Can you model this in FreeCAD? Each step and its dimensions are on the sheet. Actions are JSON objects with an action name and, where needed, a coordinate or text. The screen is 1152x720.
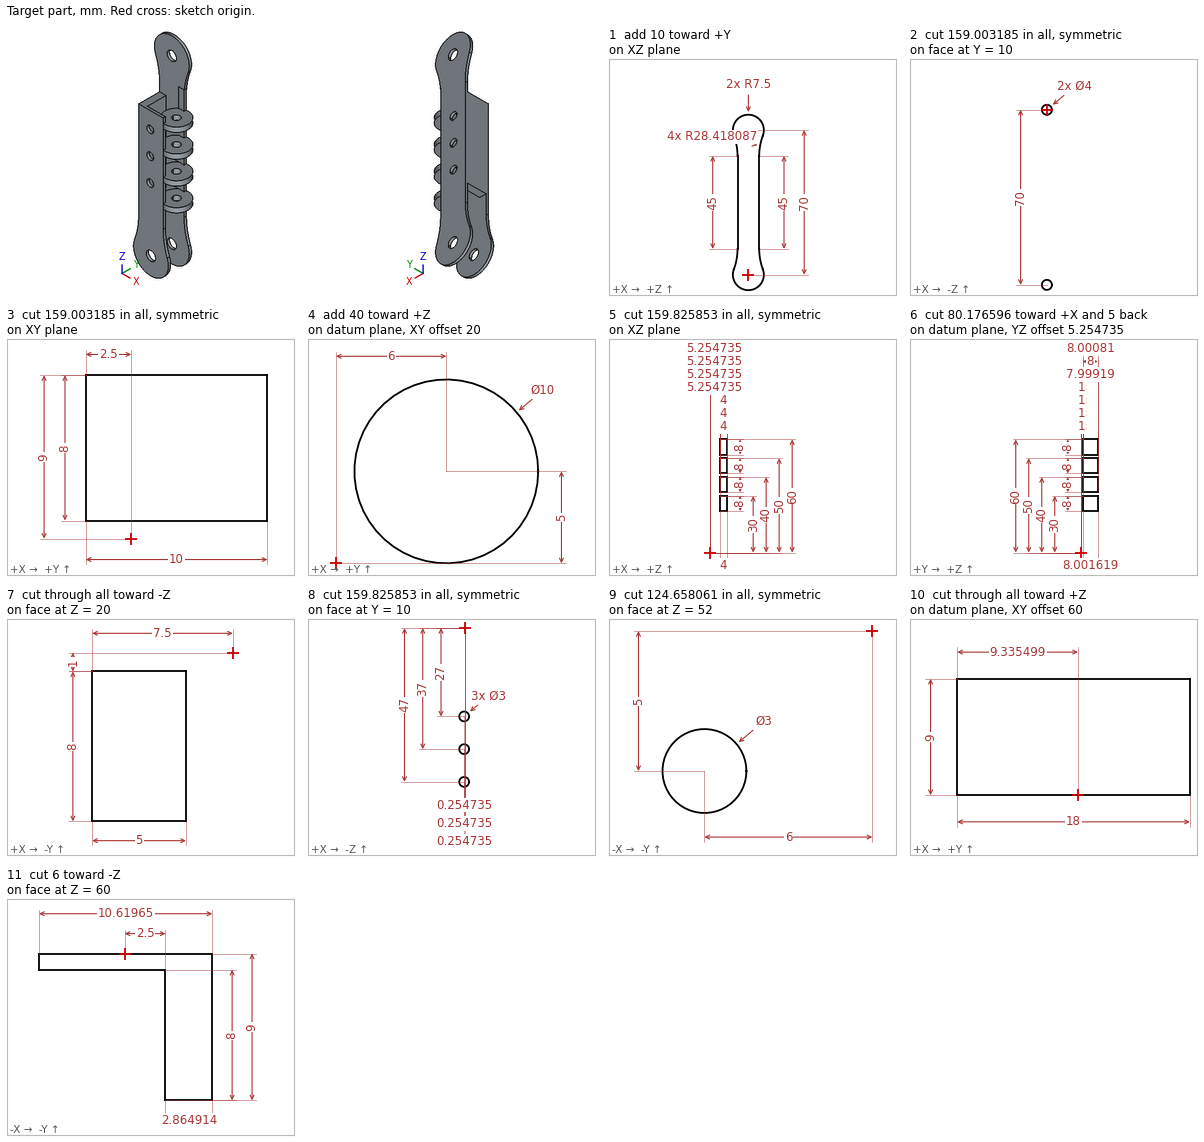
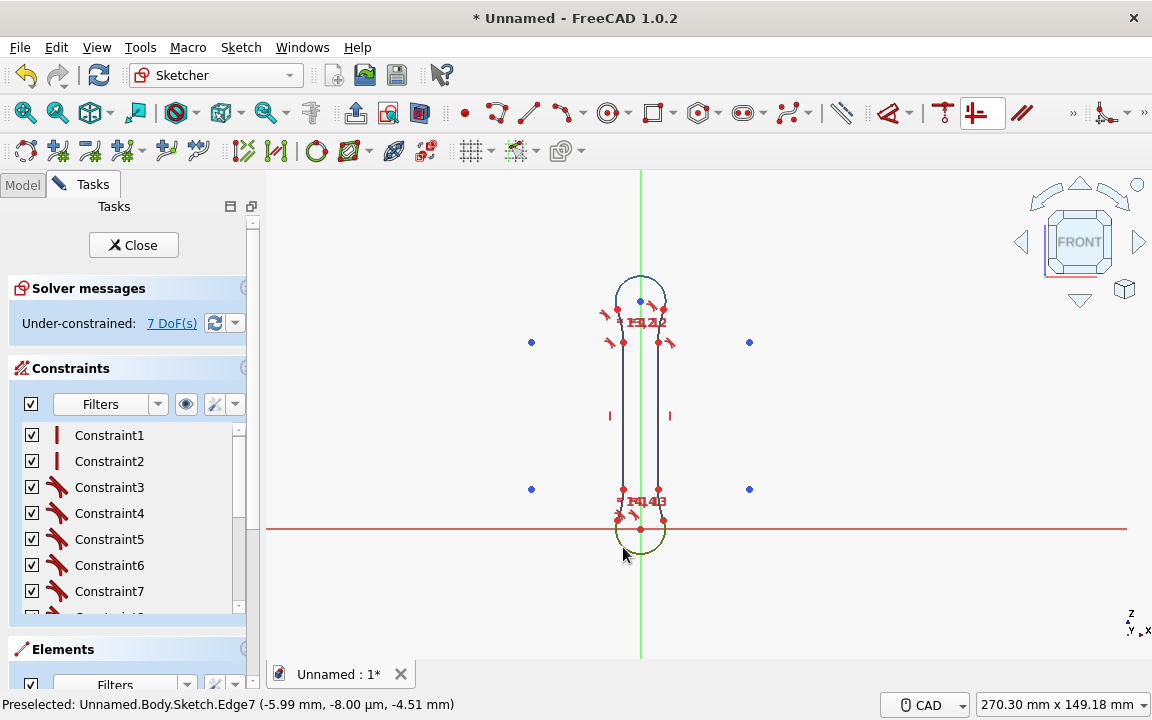
{"action": "key", "text": "e"}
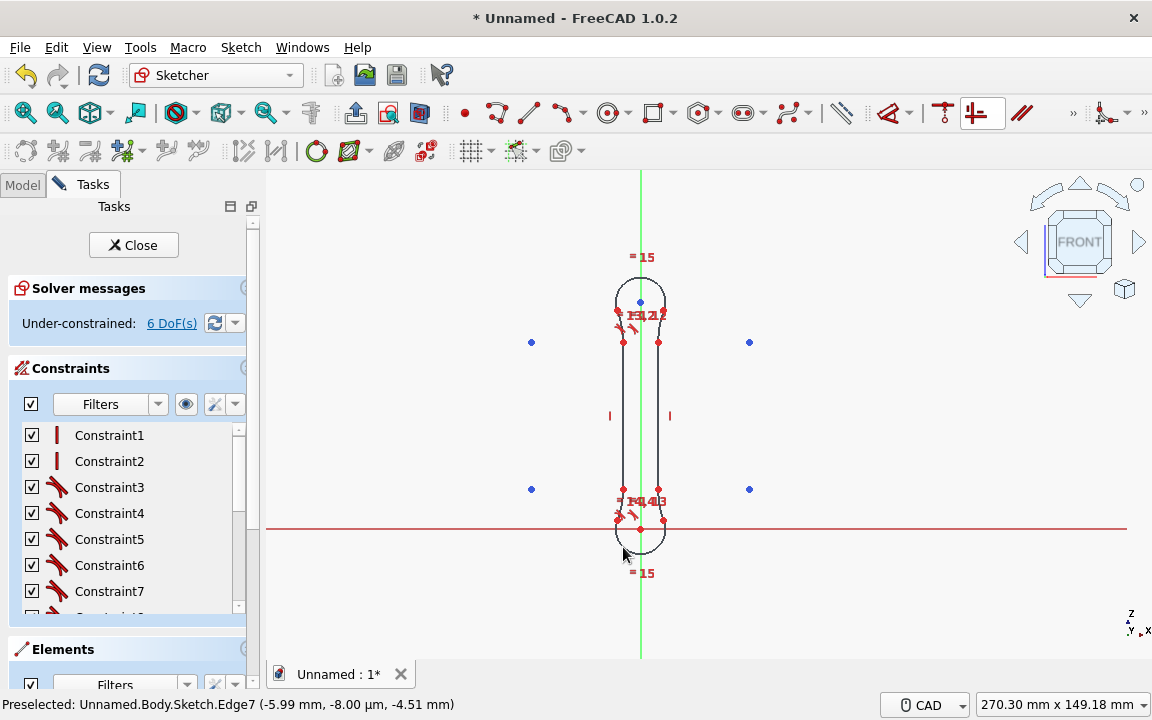
{"action": "left_click", "coordinate": [641, 302]}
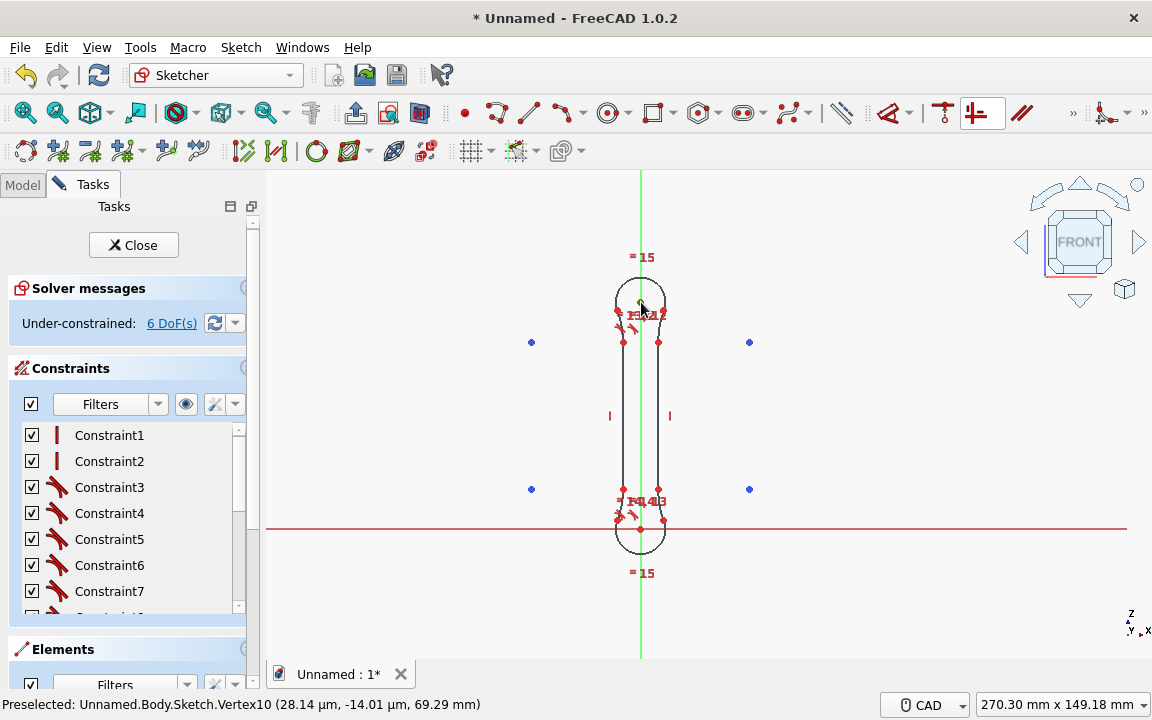
{"action": "left_click", "coordinate": [641, 600]}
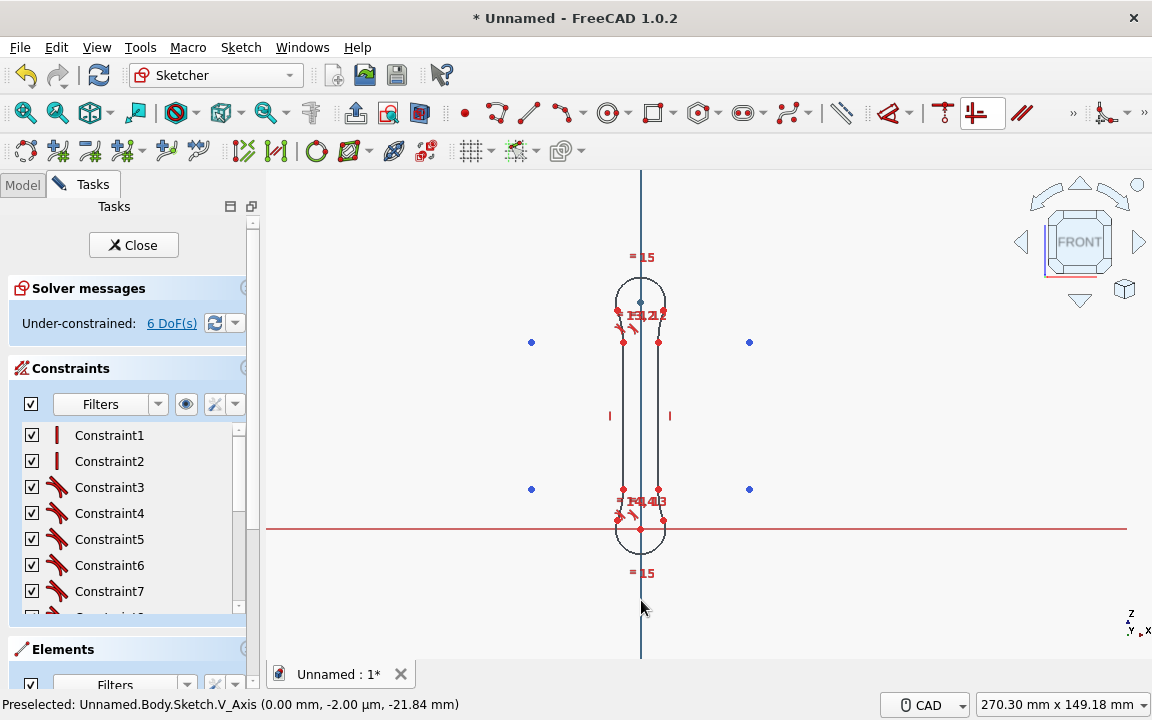
{"action": "left_click", "coordinate": [944, 114]}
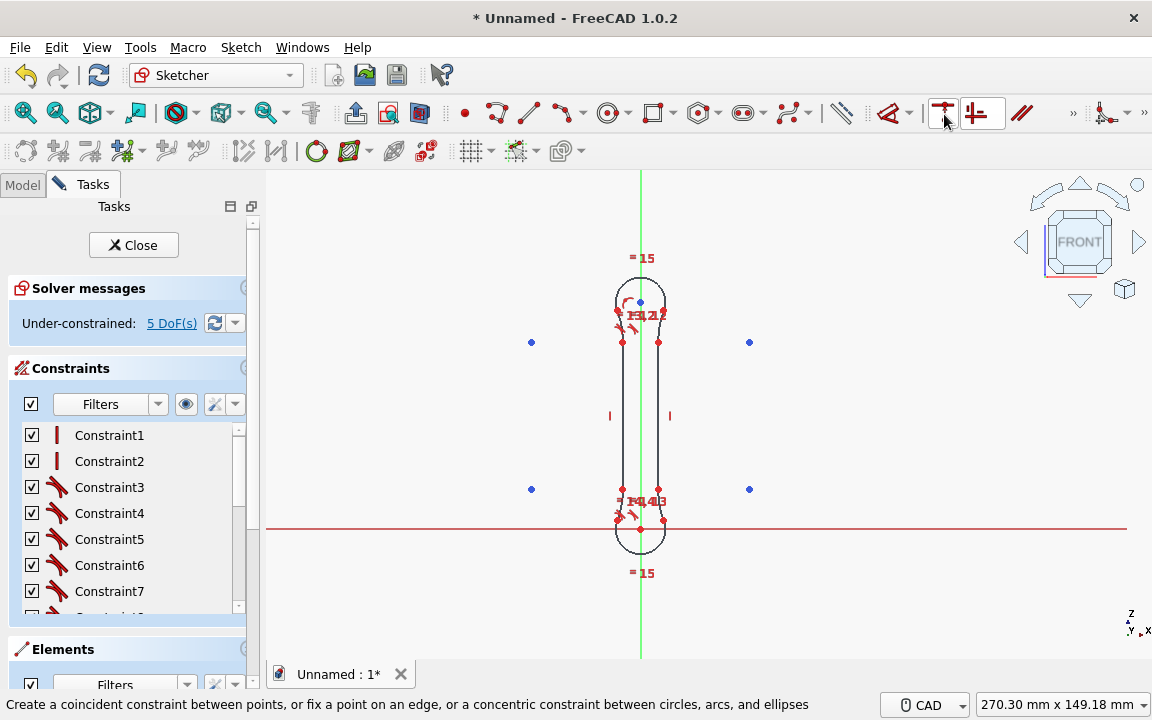
{"action": "left_click", "coordinate": [888, 114]}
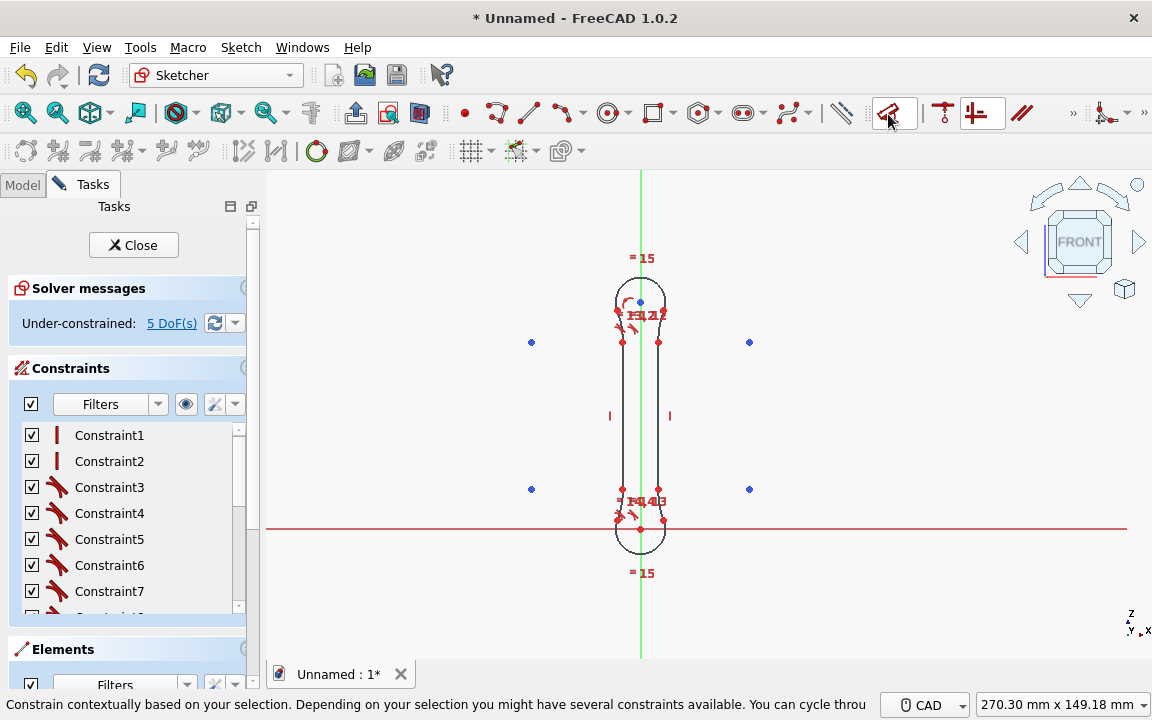
{"action": "scroll", "coordinate": [622, 333], "scroll_direction": "up", "scroll_amount": 2}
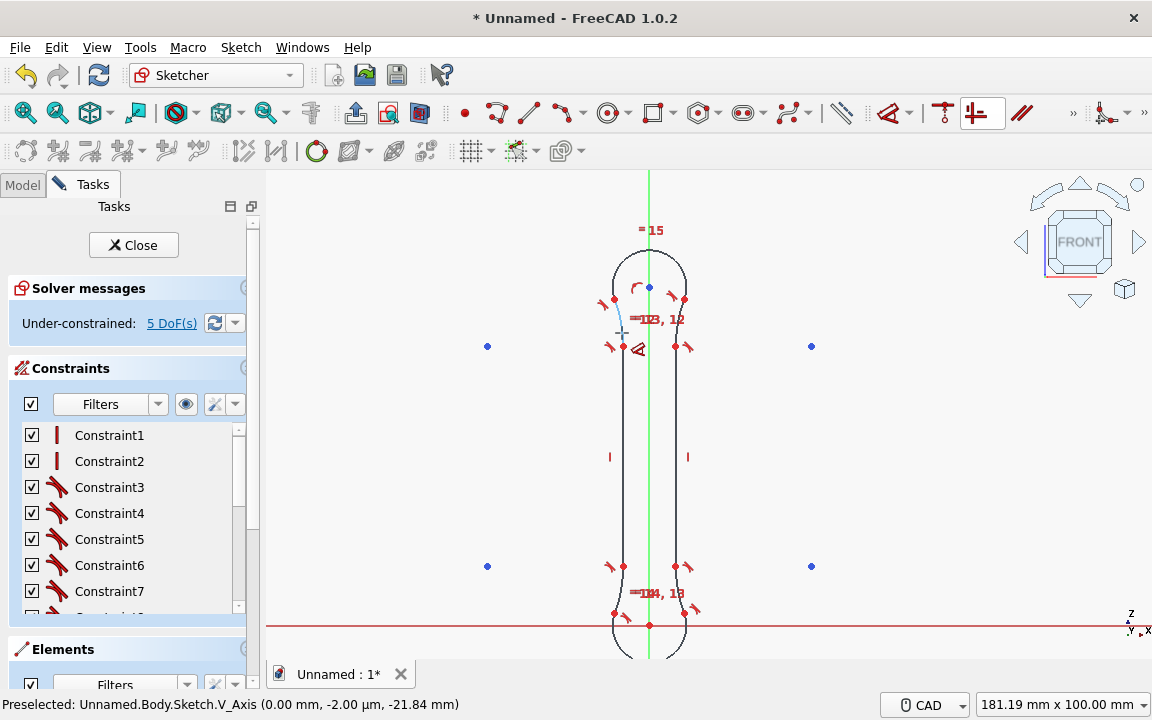
{"action": "left_click", "coordinate": [622, 332]}
{"action": "left_click", "coordinate": [592, 477]}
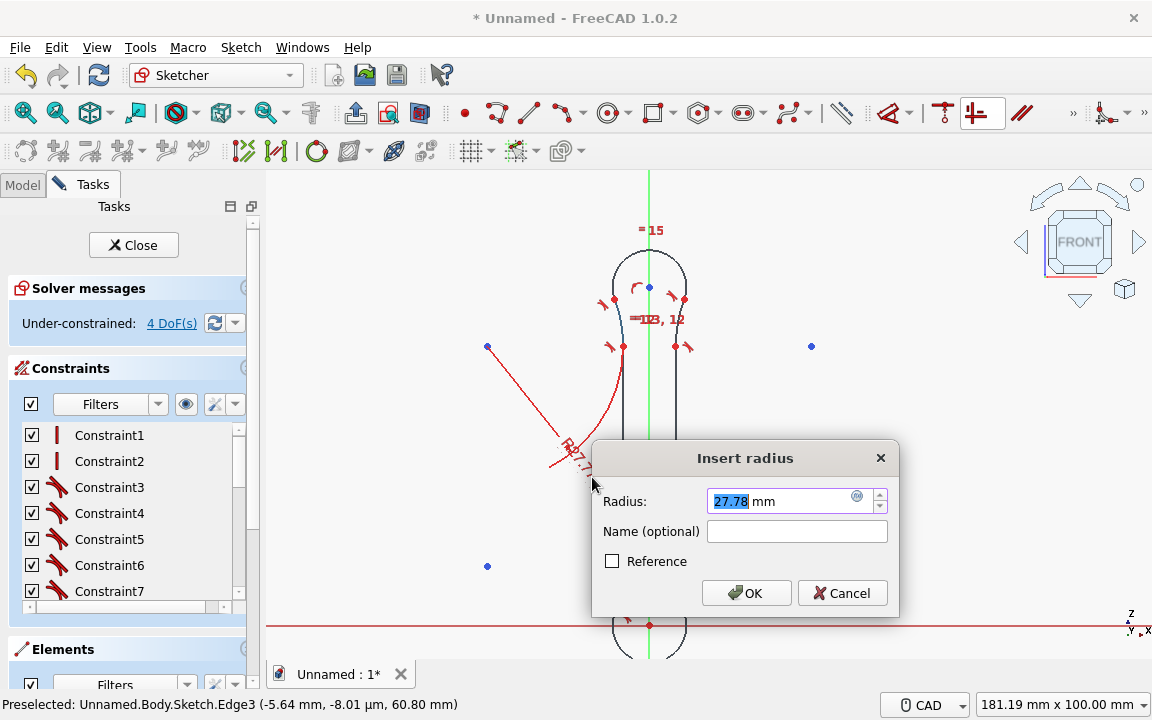
{"action": "type", "text": "28.418087"}
{"action": "key", "text": "Return"}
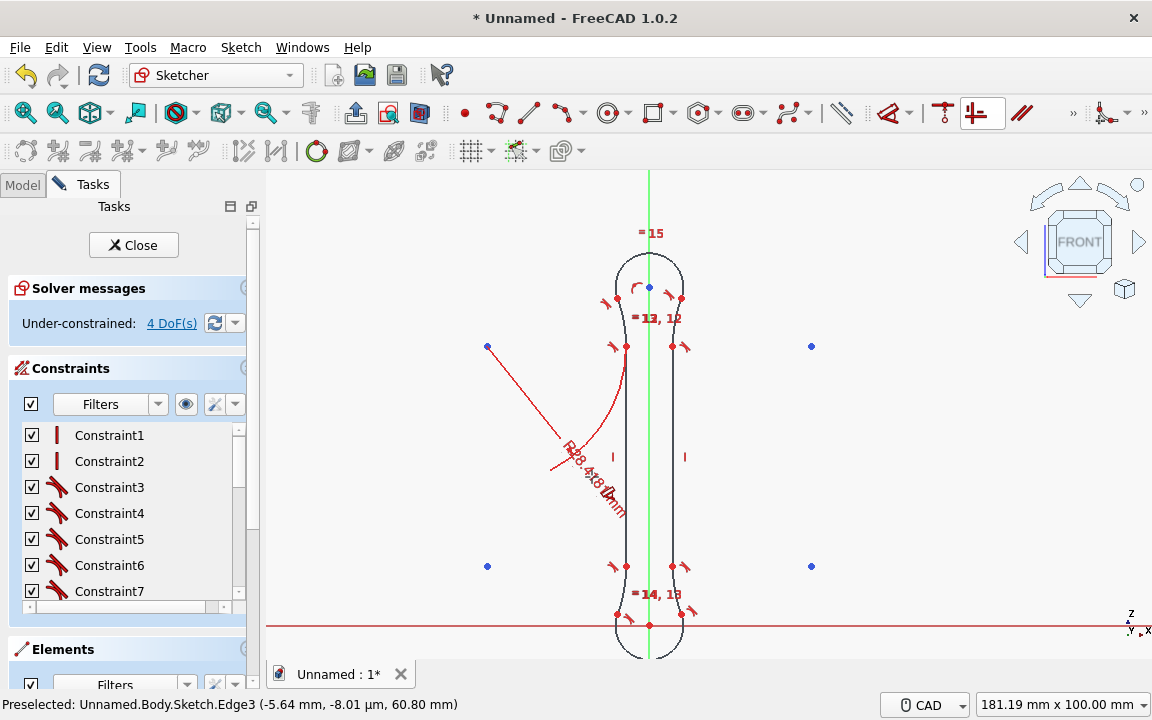
{"action": "left_click", "coordinate": [673, 263]}
{"action": "left_click", "coordinate": [695, 240]}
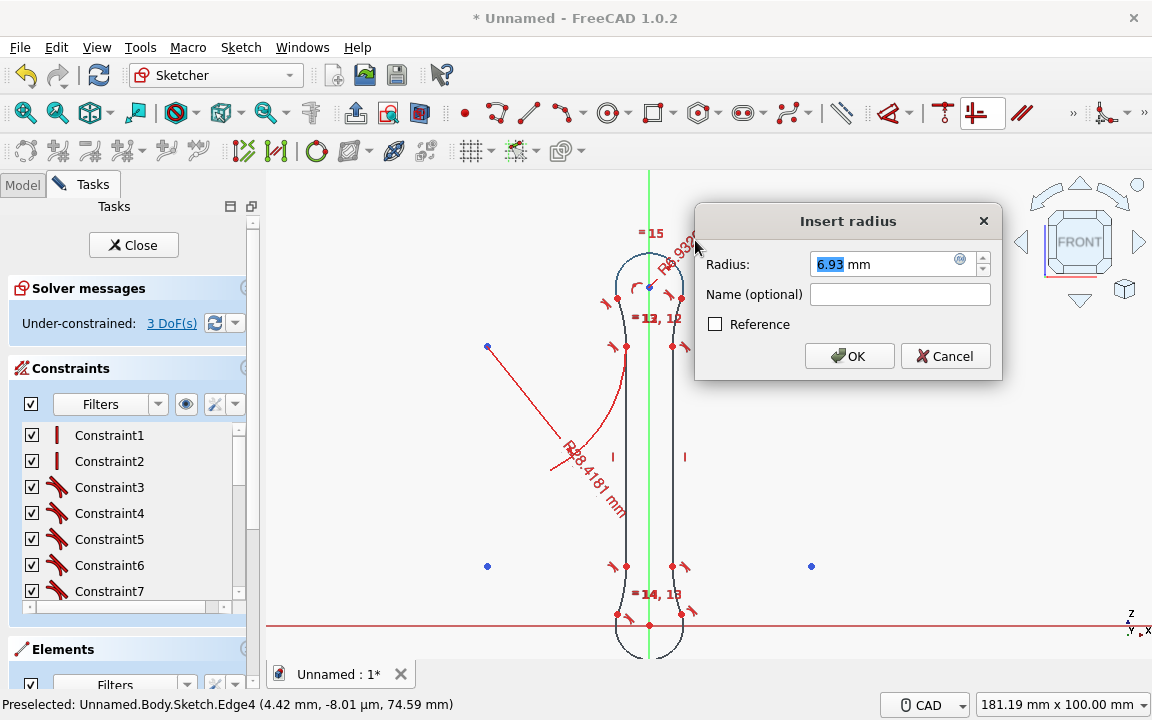
{"action": "type", "text": "7.5"}
{"action": "key", "text": "Return"}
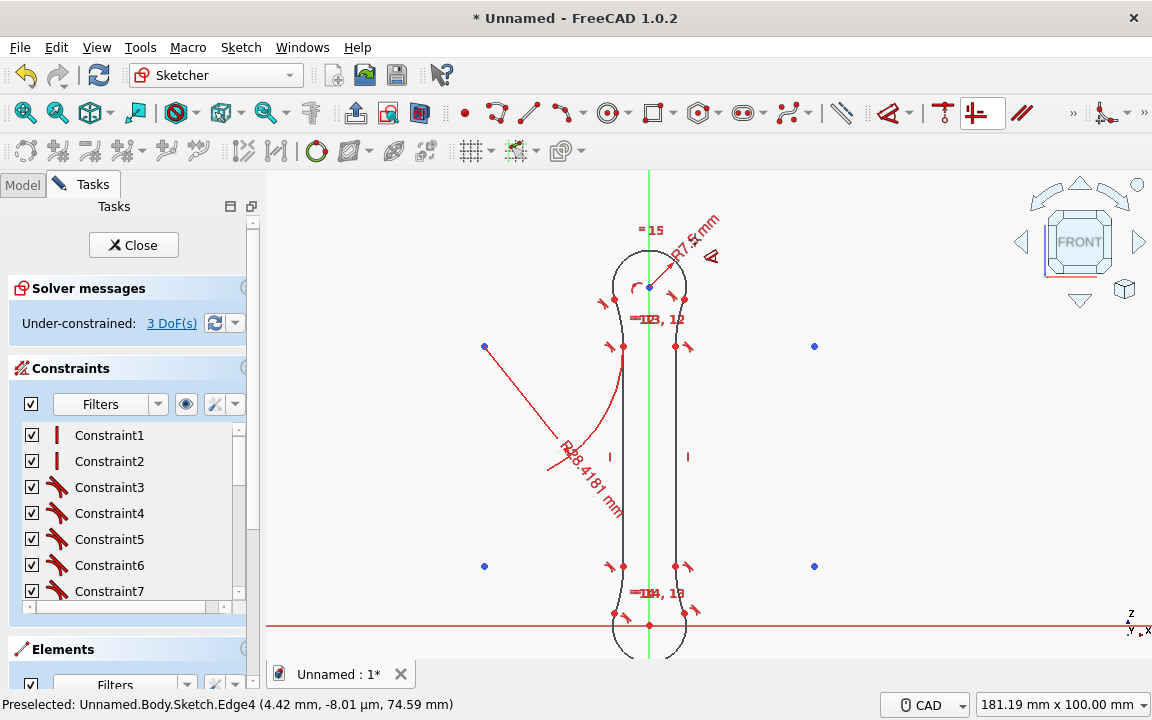
{"action": "left_click", "coordinate": [623, 500]}
{"action": "left_click", "coordinate": [589, 457]}